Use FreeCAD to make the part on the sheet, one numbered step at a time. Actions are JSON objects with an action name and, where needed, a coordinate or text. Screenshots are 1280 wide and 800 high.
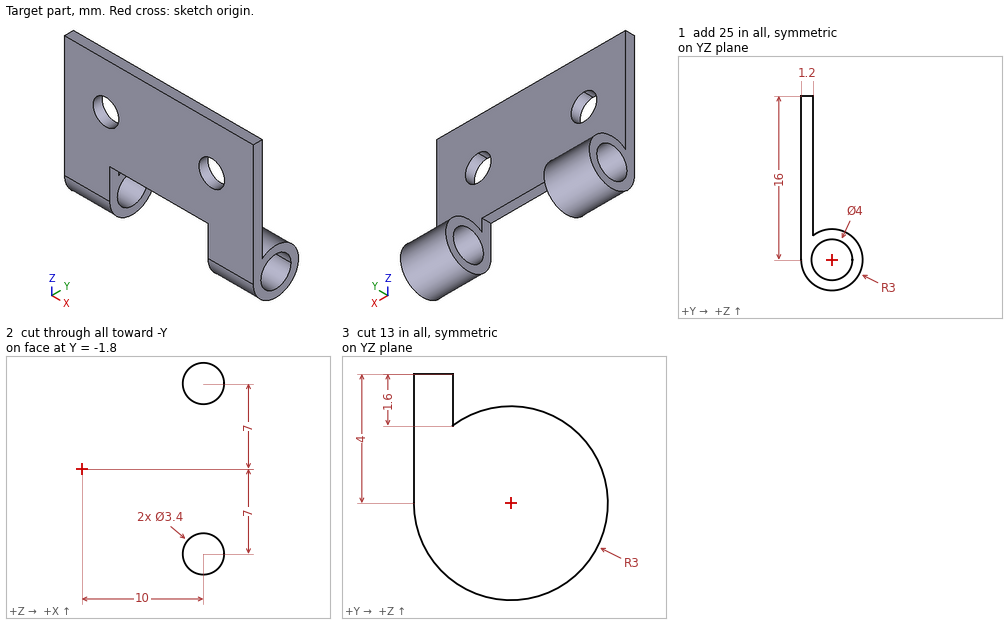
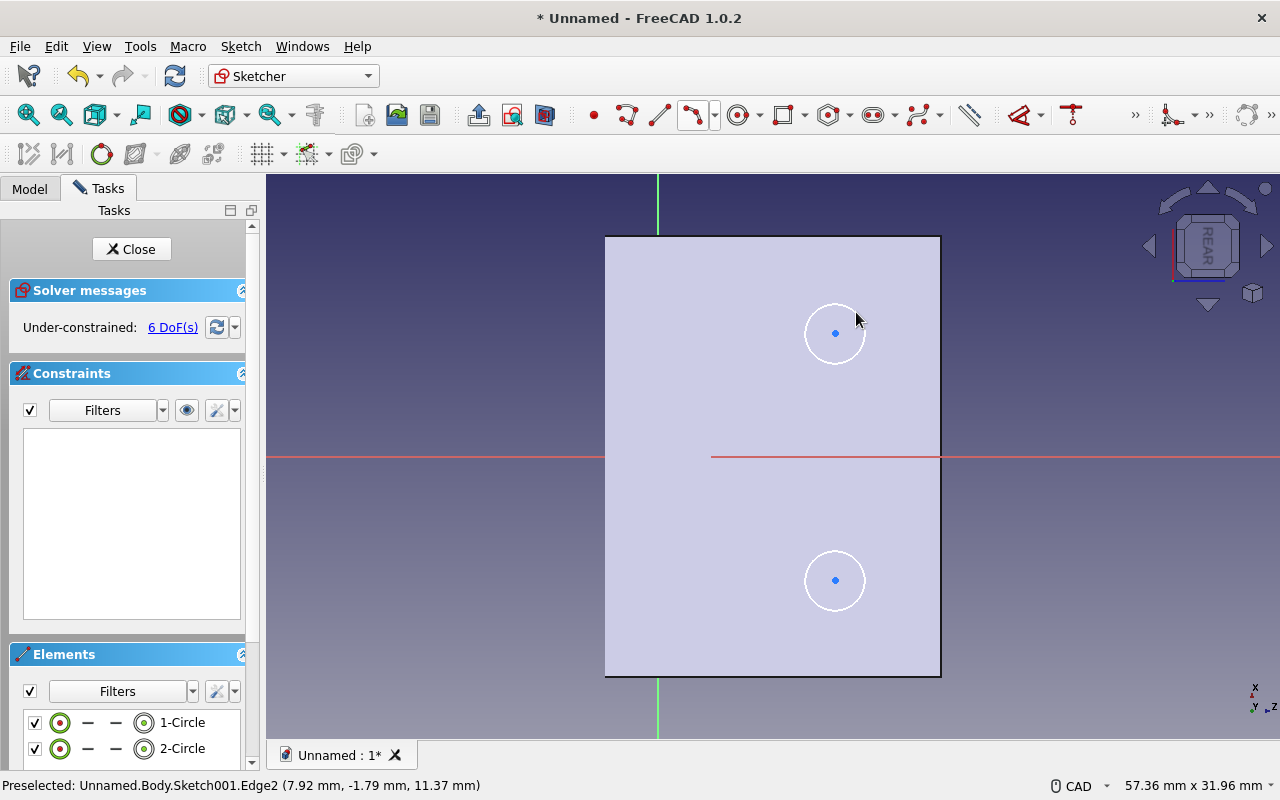
{"action": "left_click", "coordinate": [856, 560]}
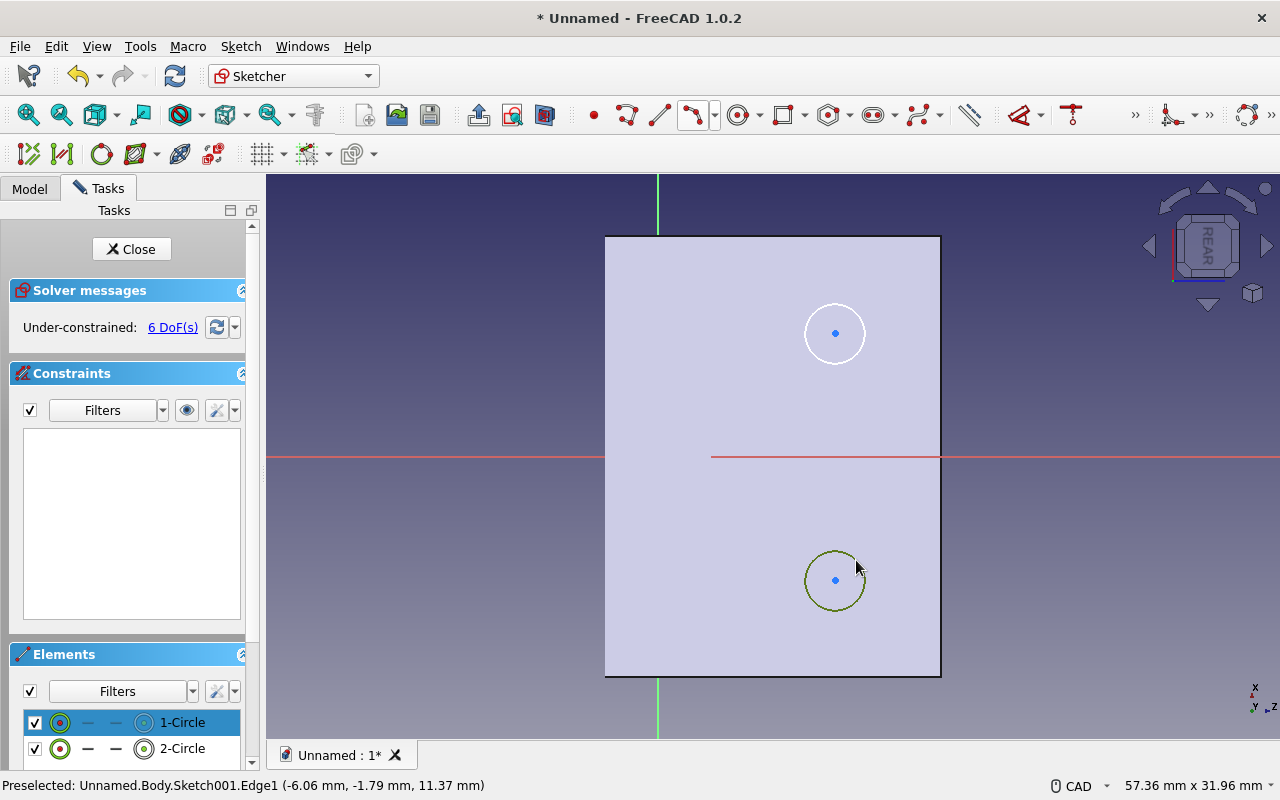
{"action": "left_click", "coordinate": [856, 313]}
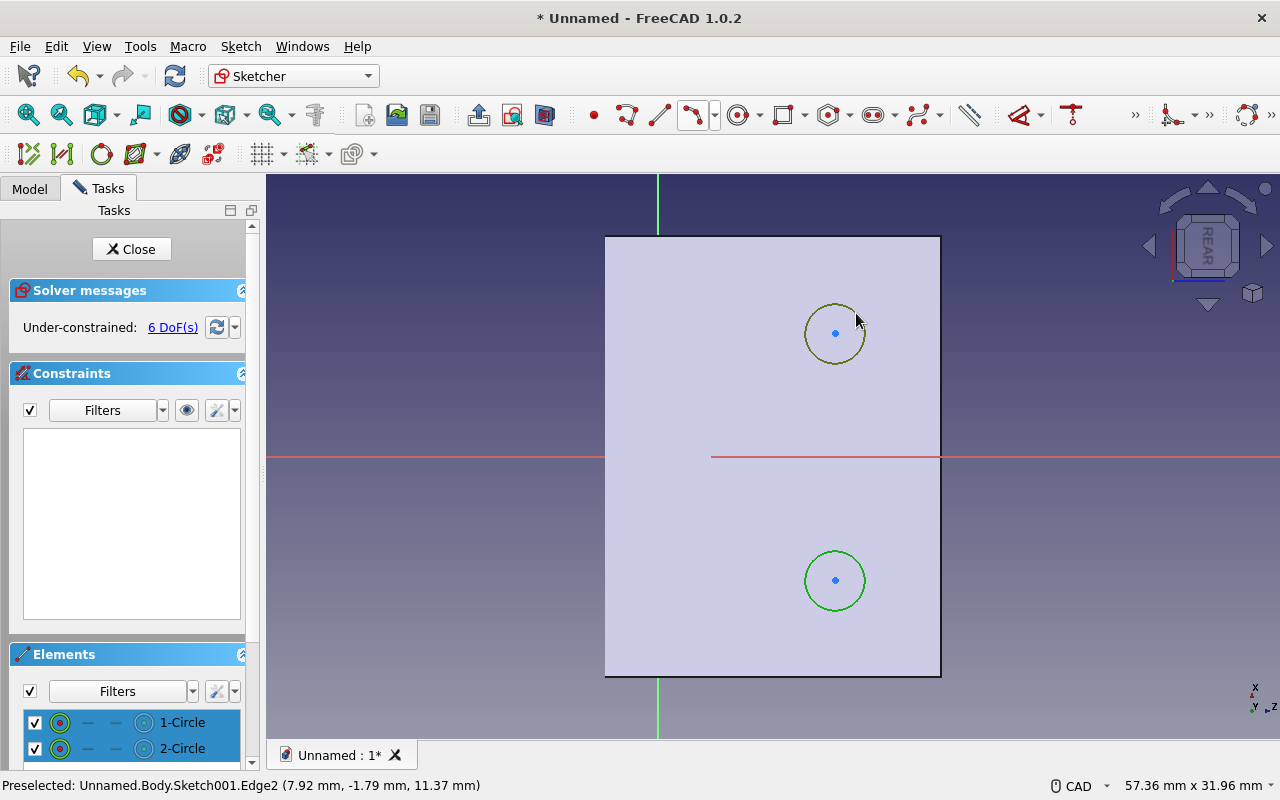
{"action": "key", "text": "e"}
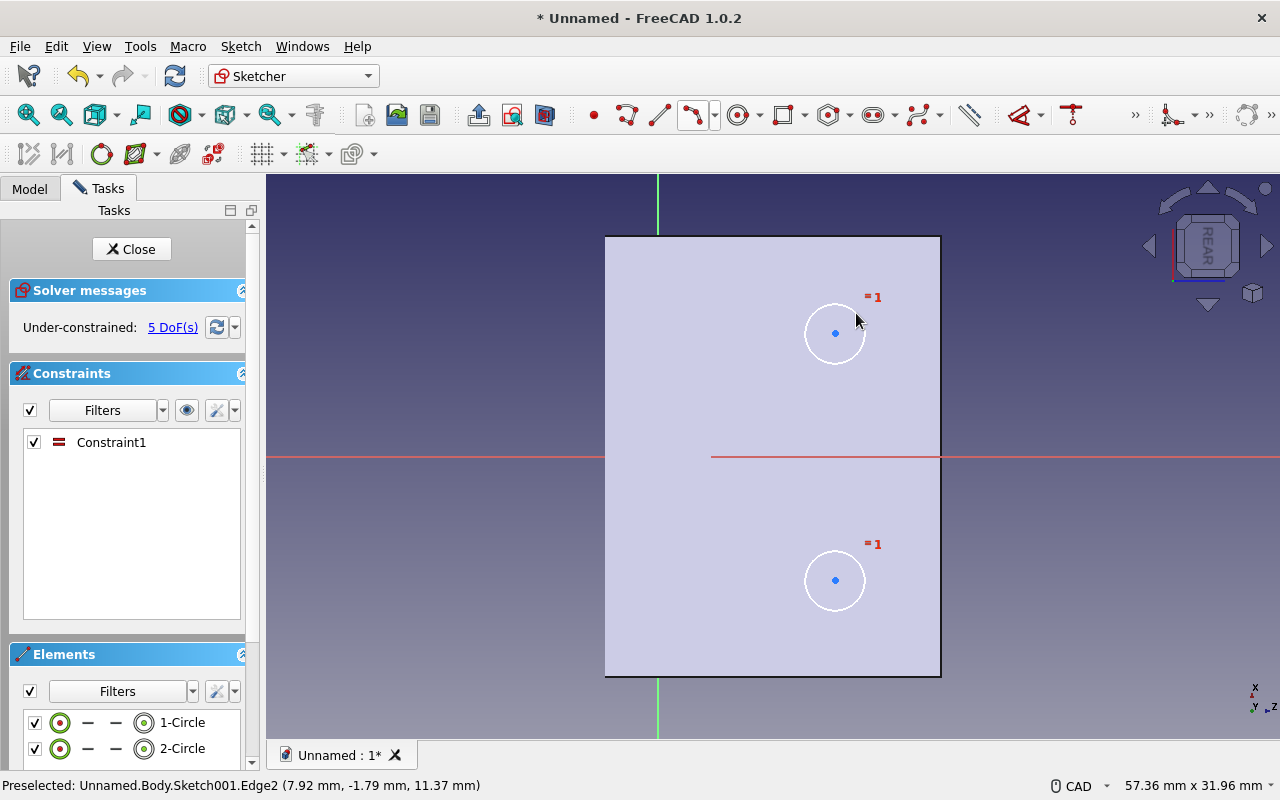
{"action": "left_click", "coordinate": [835, 581]}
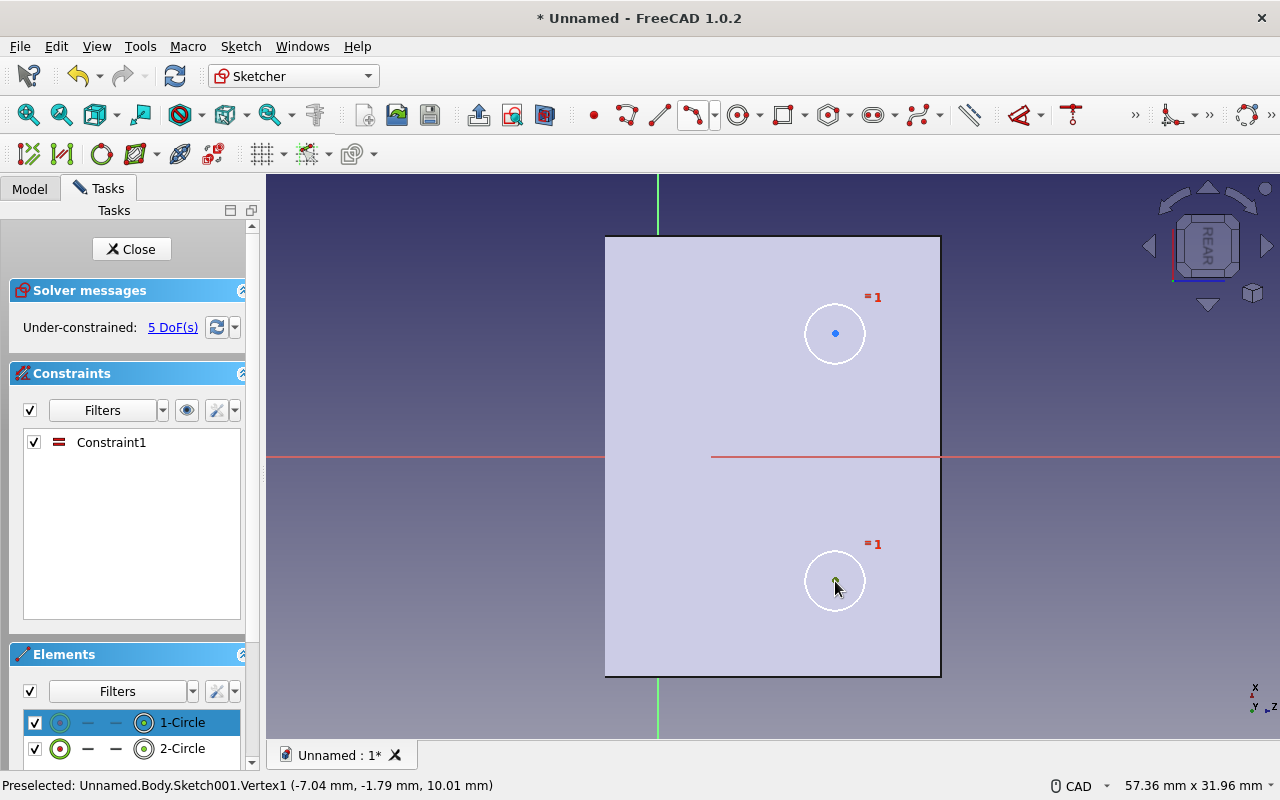
{"action": "left_click", "coordinate": [835, 334]}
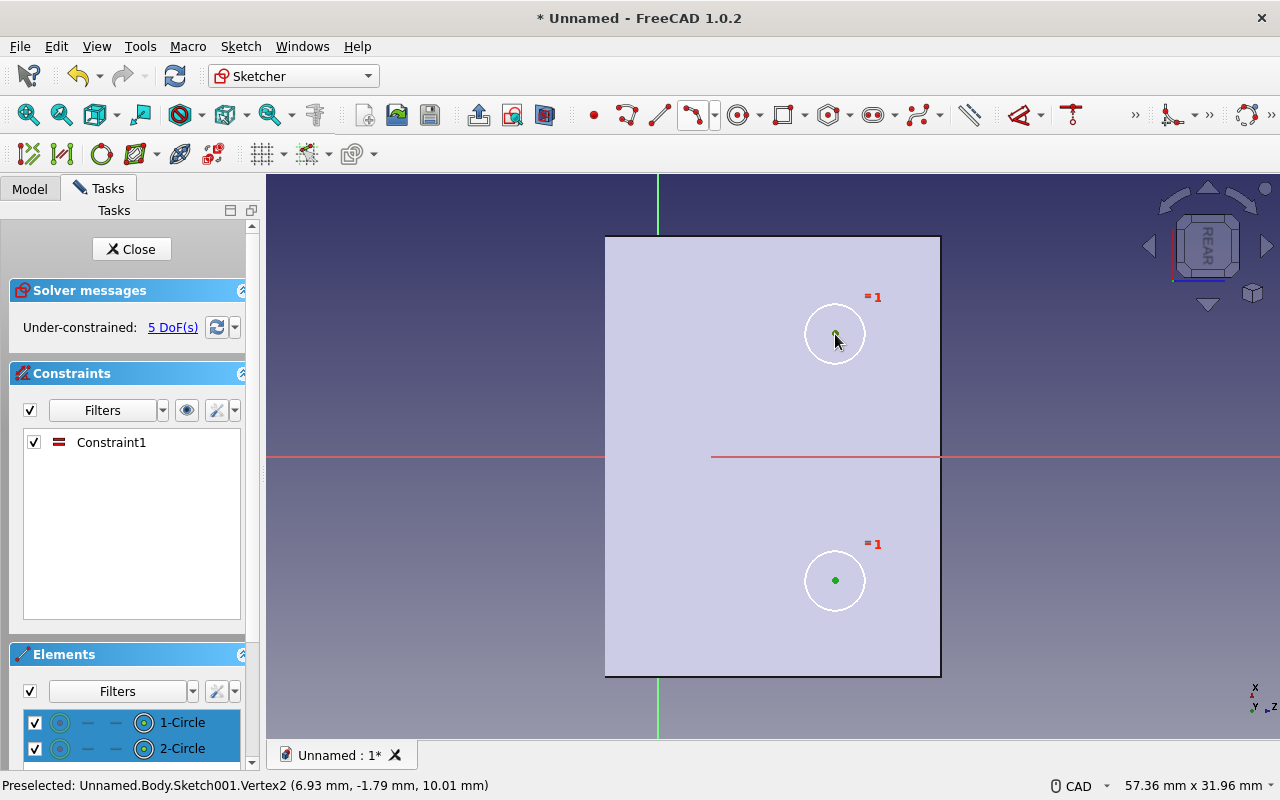
{"action": "key", "text": "v"}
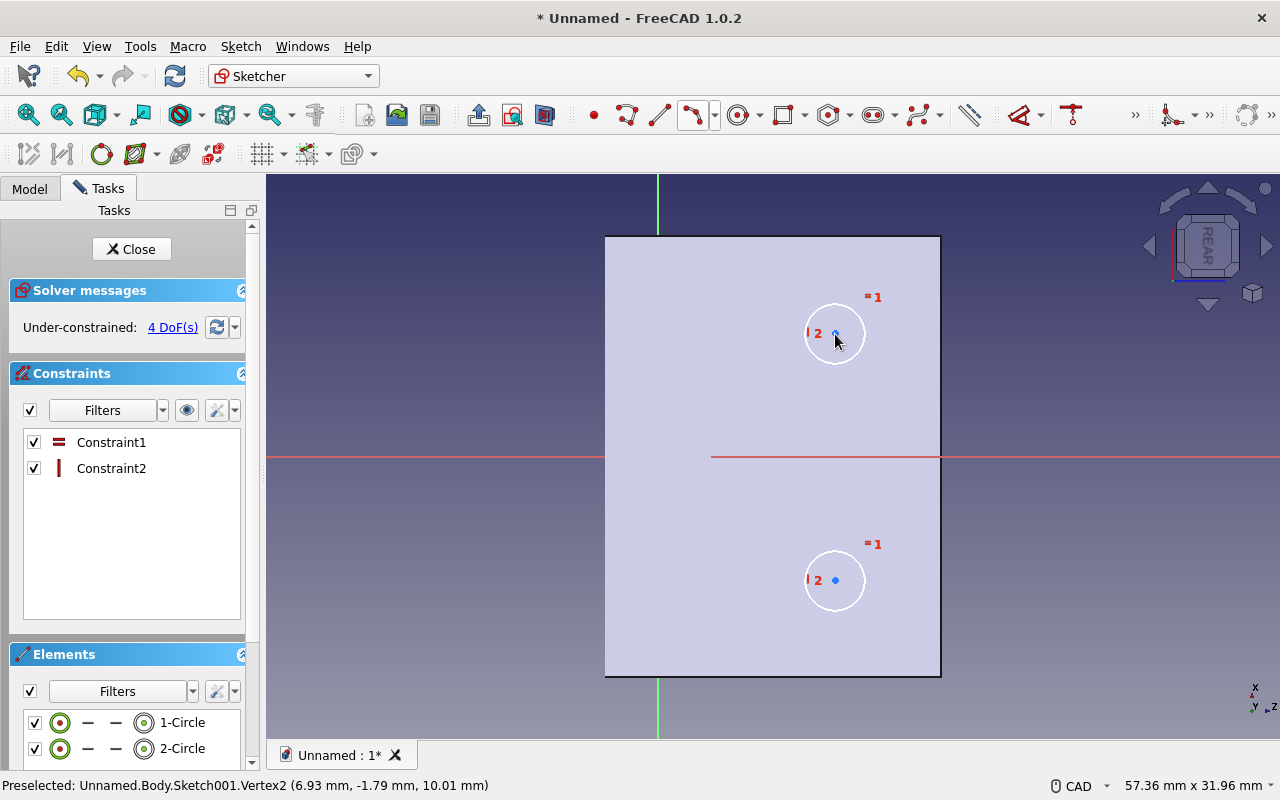
{"action": "left_click", "coordinate": [1018, 116]}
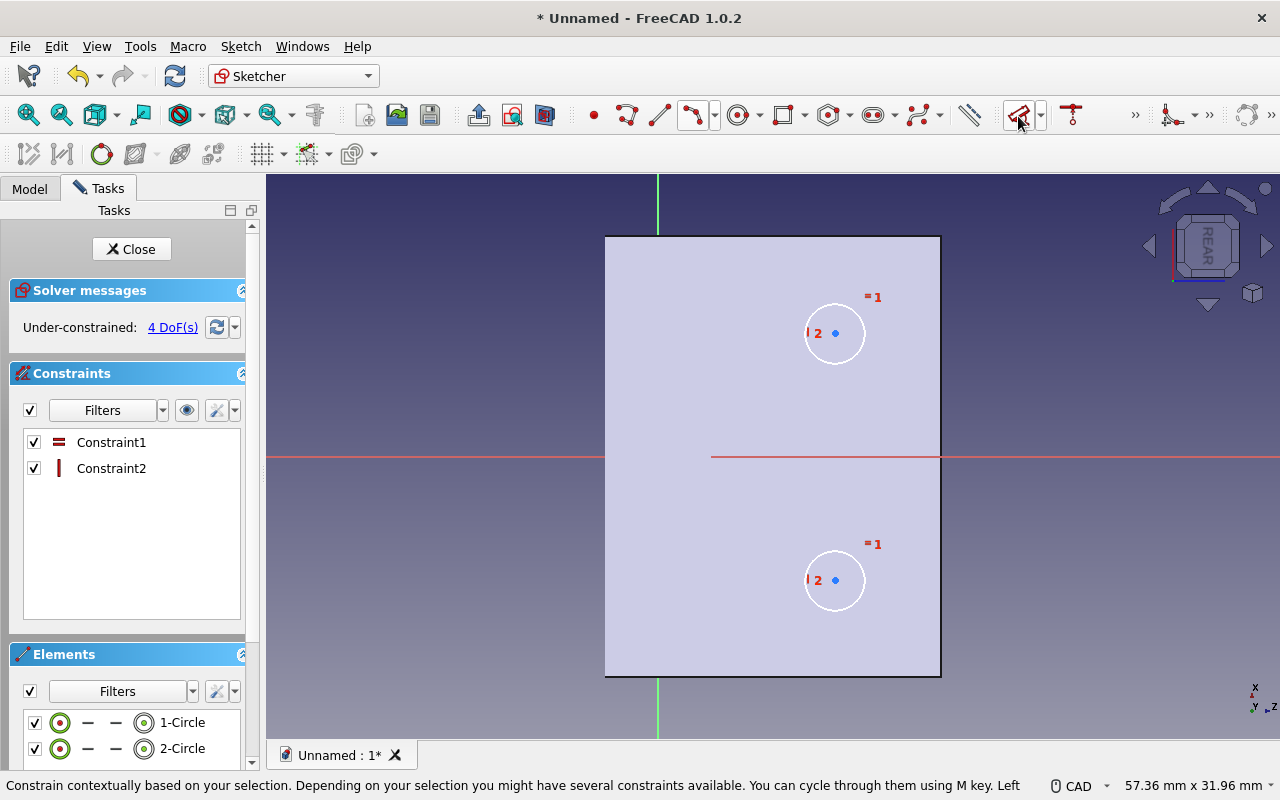
{"action": "left_click", "coordinate": [856, 560]}
{"action": "left_click", "coordinate": [879, 537]}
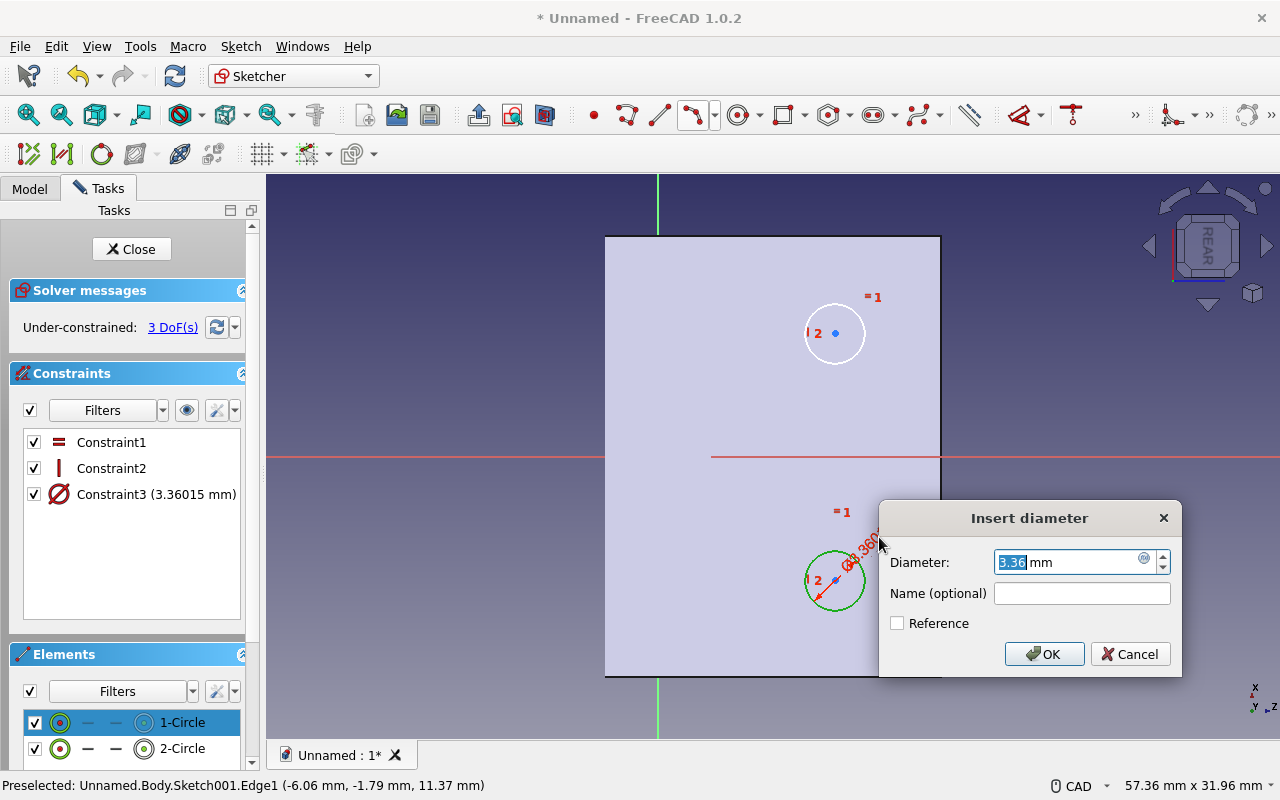
{"action": "type", "text": "3.4"}
{"action": "key", "text": "Return"}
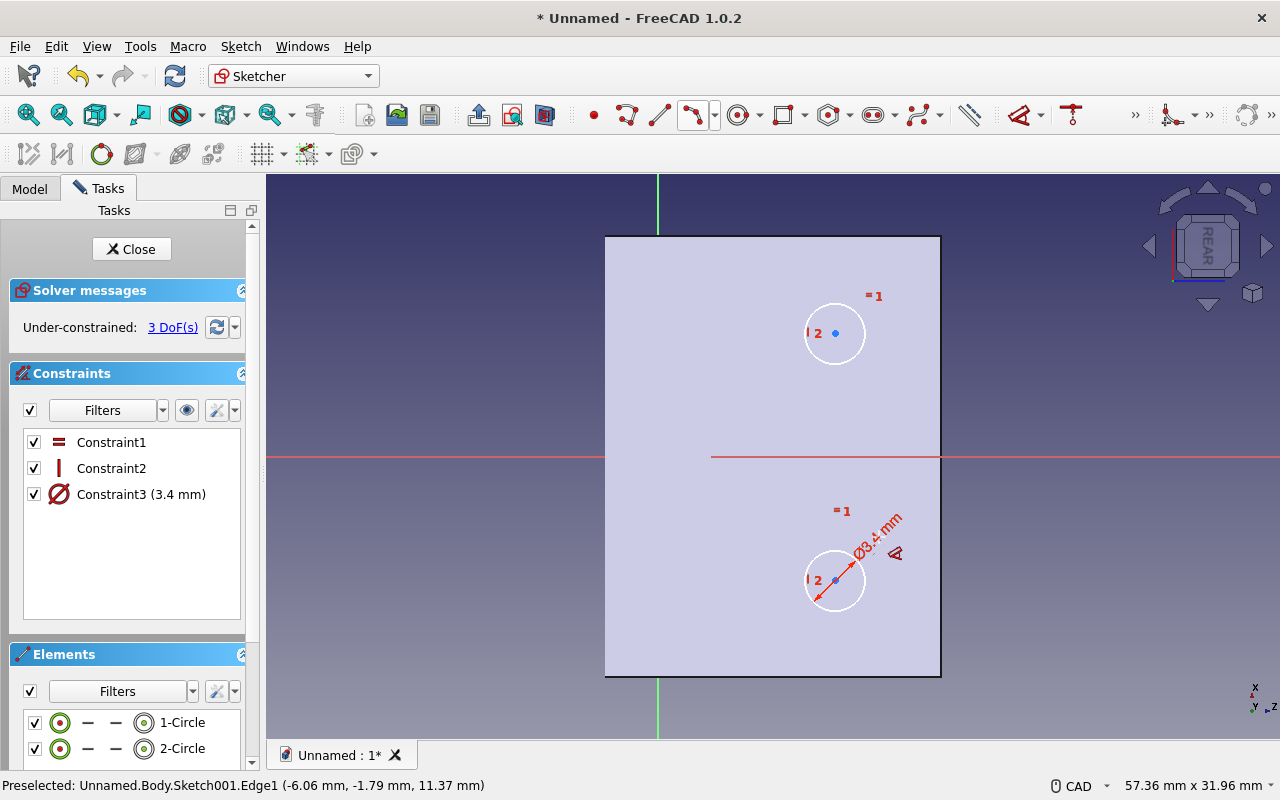
{"action": "left_click", "coordinate": [835, 581]}
{"action": "left_click", "coordinate": [624, 519]}